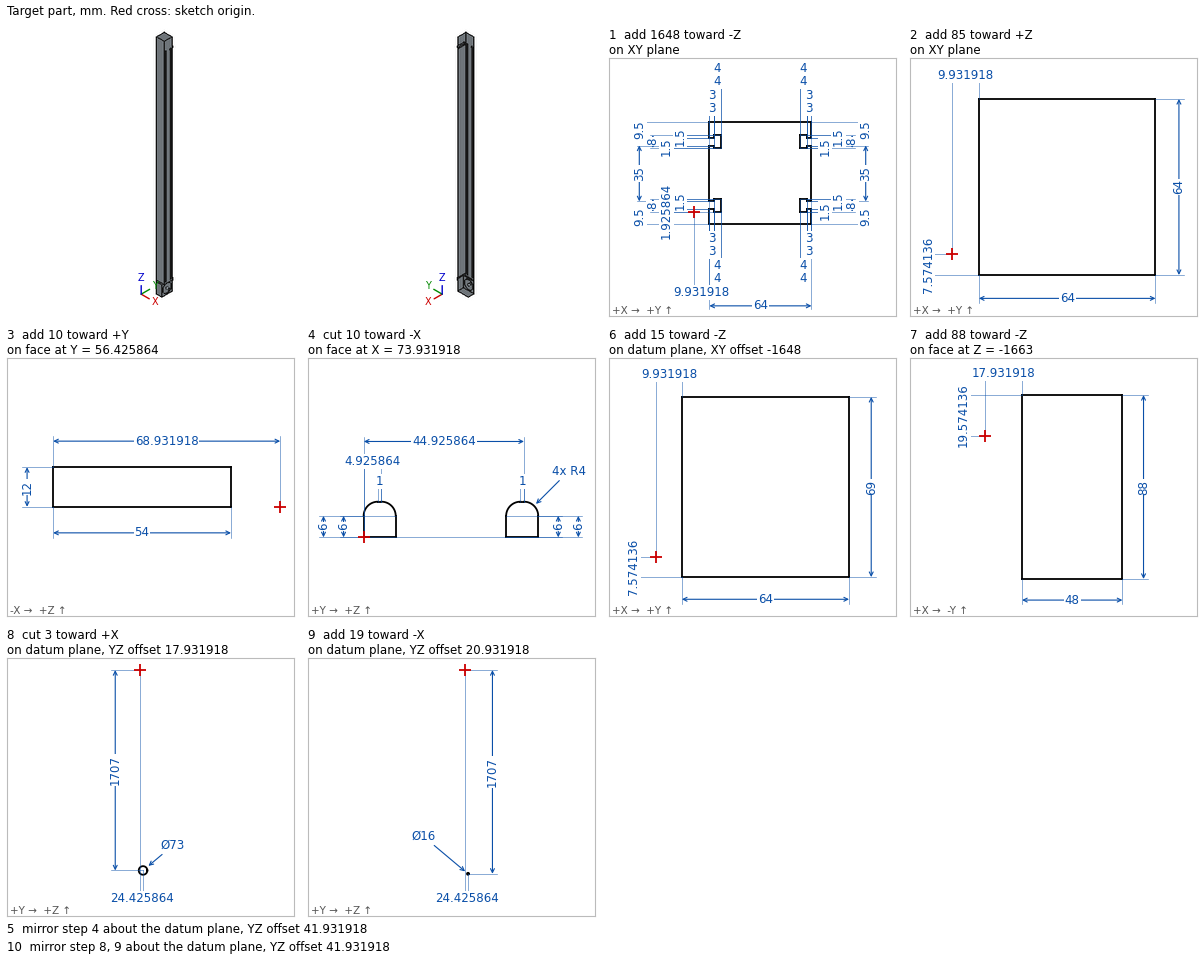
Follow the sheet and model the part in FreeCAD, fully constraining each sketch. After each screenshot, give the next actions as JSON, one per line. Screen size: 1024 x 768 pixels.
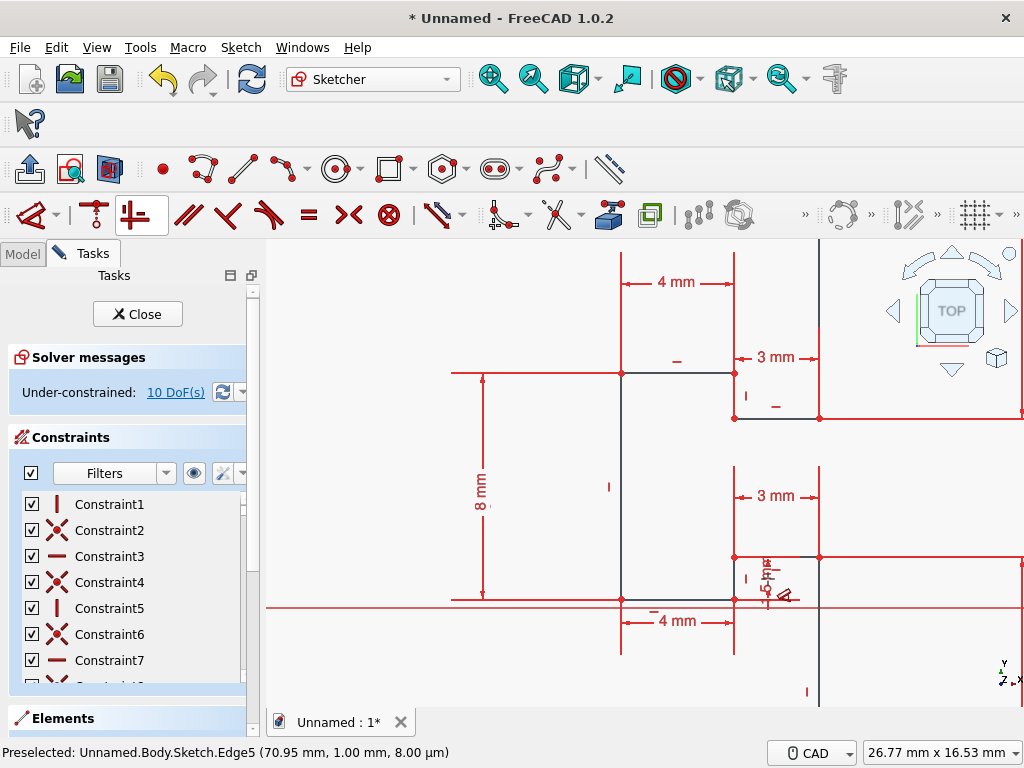
{"action": "left_click", "coordinate": [734, 387]}
{"action": "left_click", "coordinate": [768, 396]}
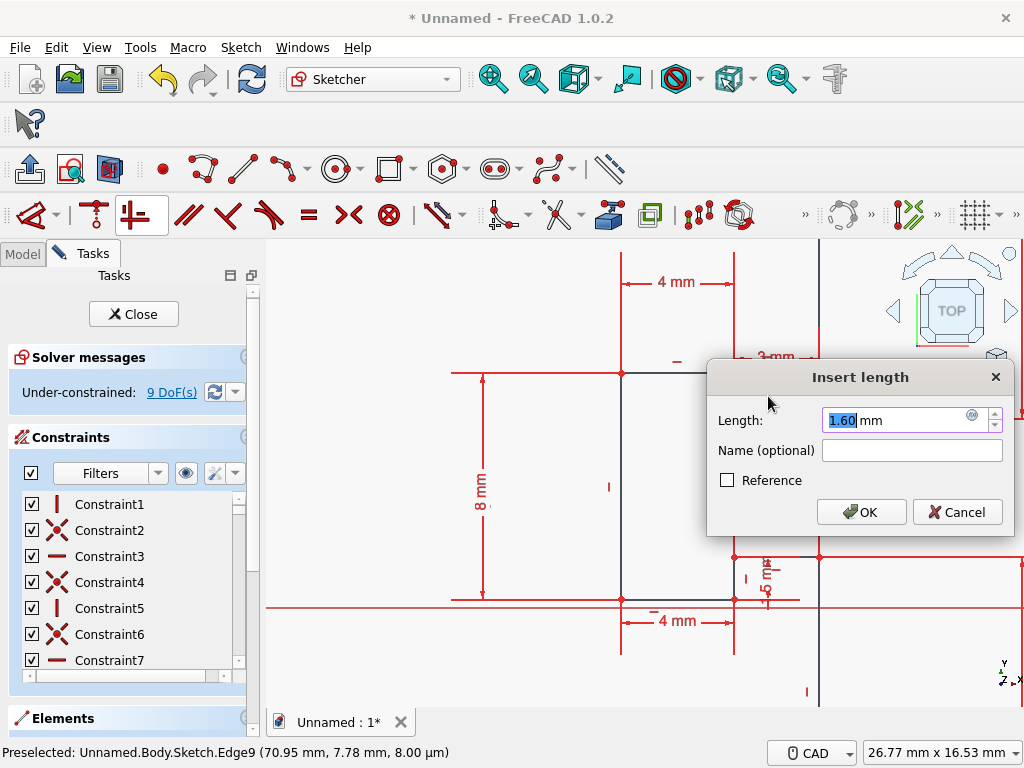
{"action": "type", "text": "1.5"}
{"action": "key", "text": "Return"}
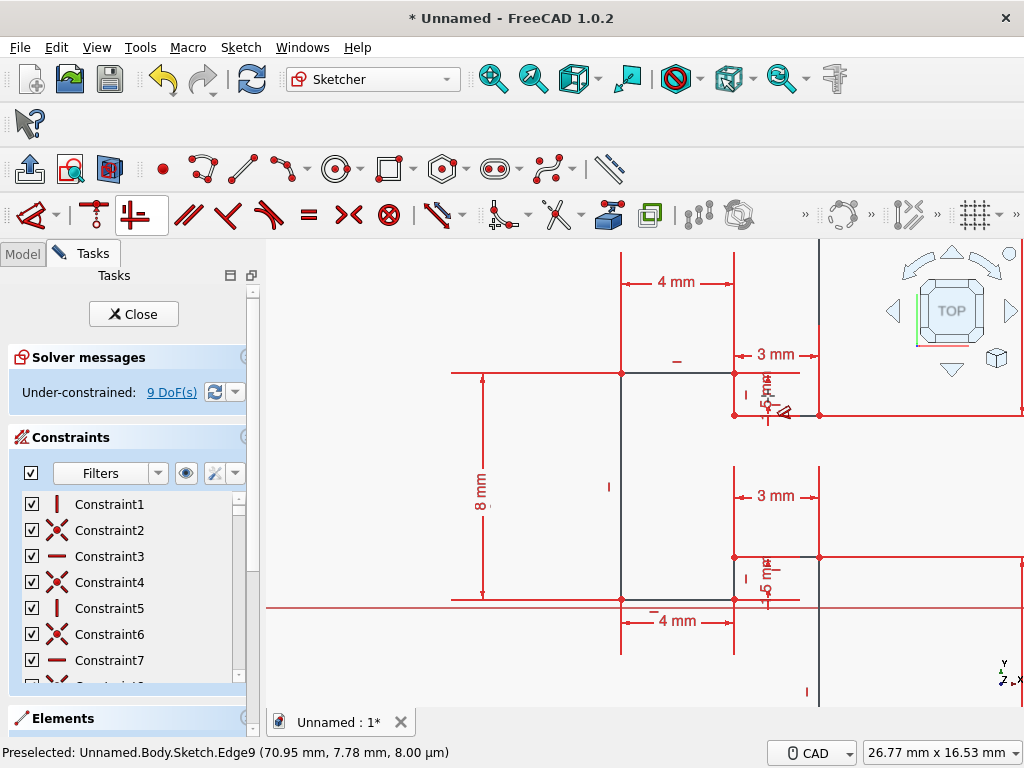
{"action": "scroll", "coordinate": [736, 583], "scroll_direction": "down", "scroll_amount": 9}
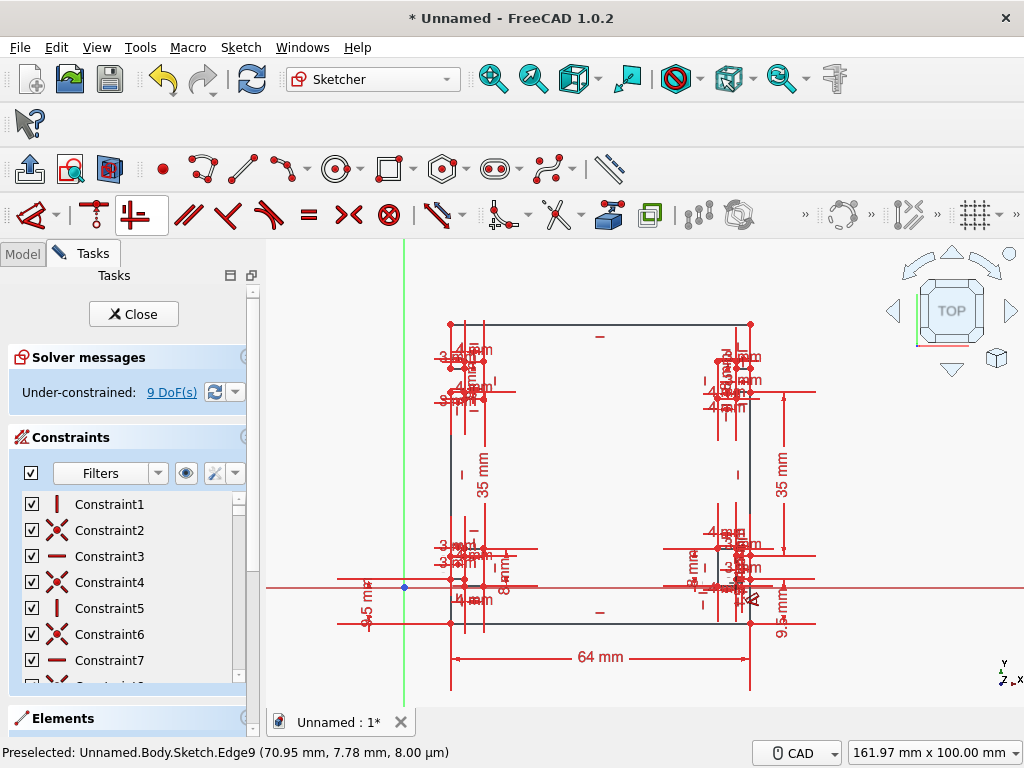
{"action": "scroll", "coordinate": [736, 394], "scroll_direction": "up", "scroll_amount": 10}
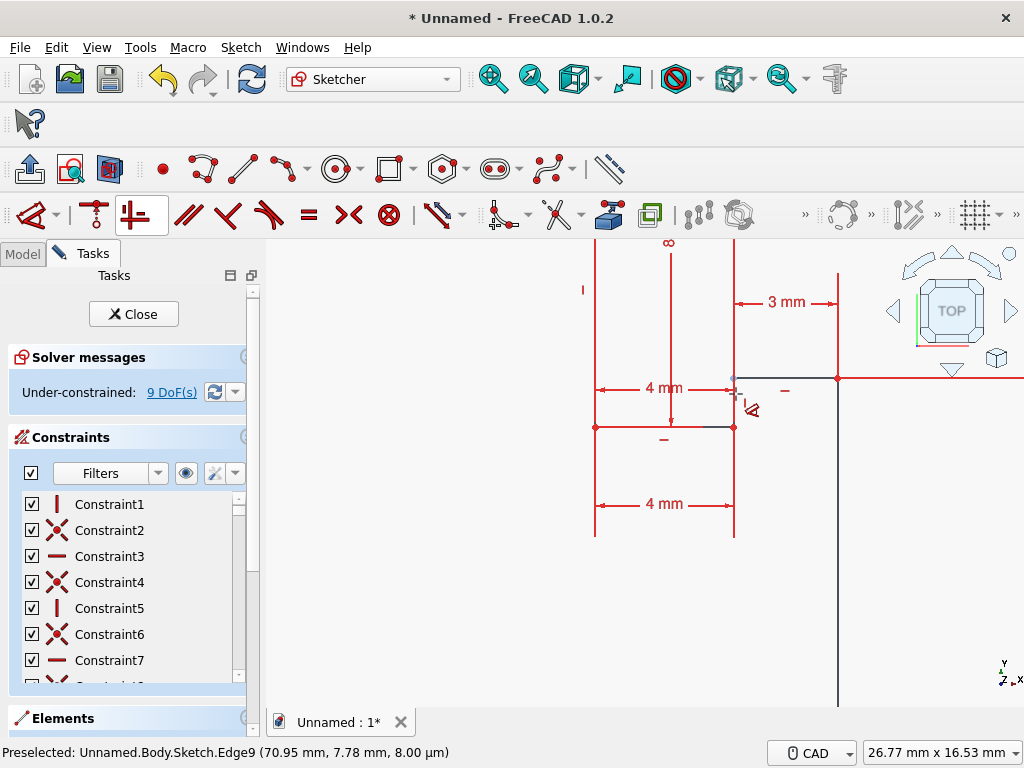
{"action": "left_click", "coordinate": [734, 393]}
{"action": "left_click", "coordinate": [768, 403]}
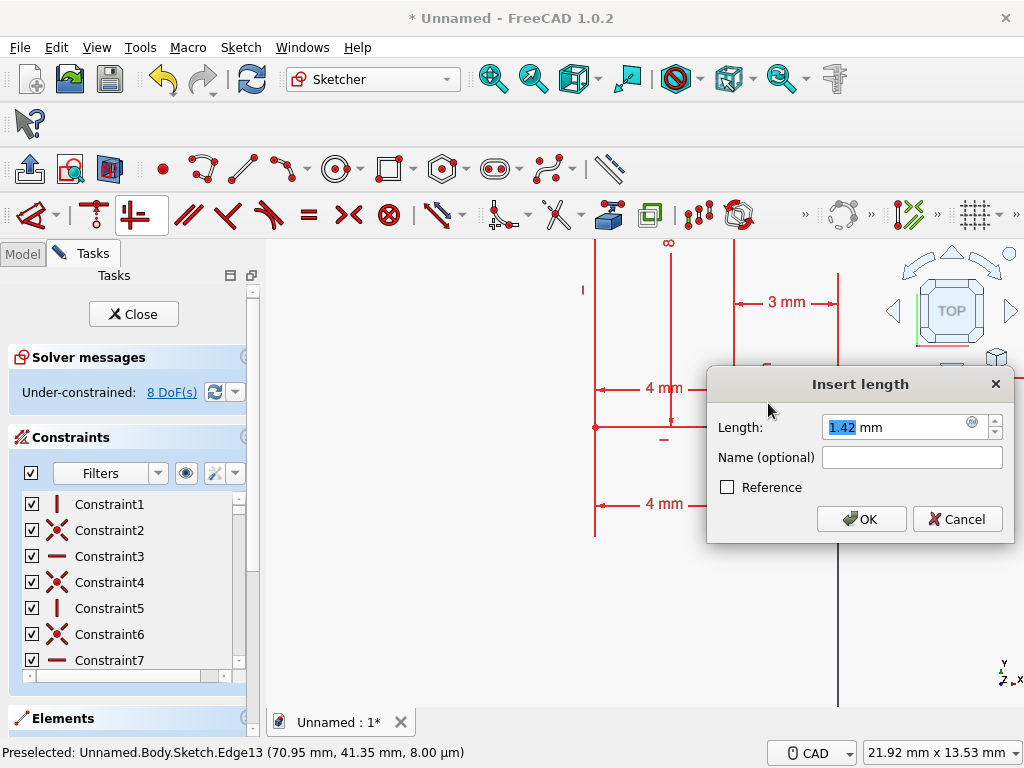
{"action": "type", "text": "1.5"}
{"action": "key", "text": "Return"}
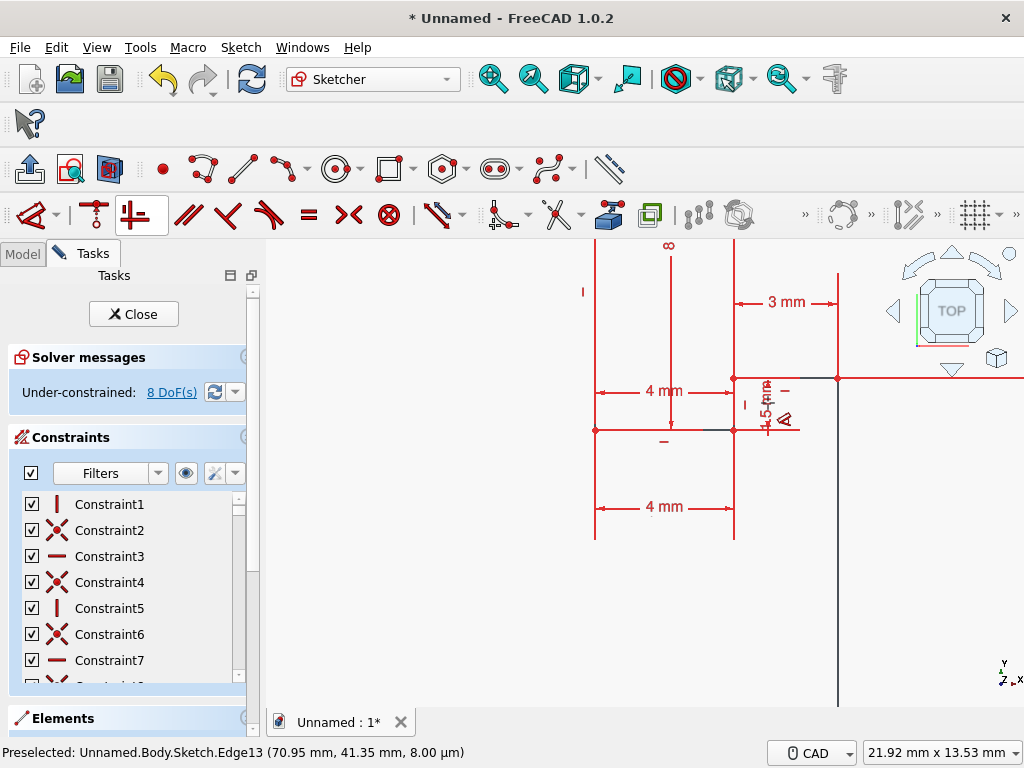
{"action": "scroll", "coordinate": [736, 394], "scroll_direction": "down", "scroll_amount": 10}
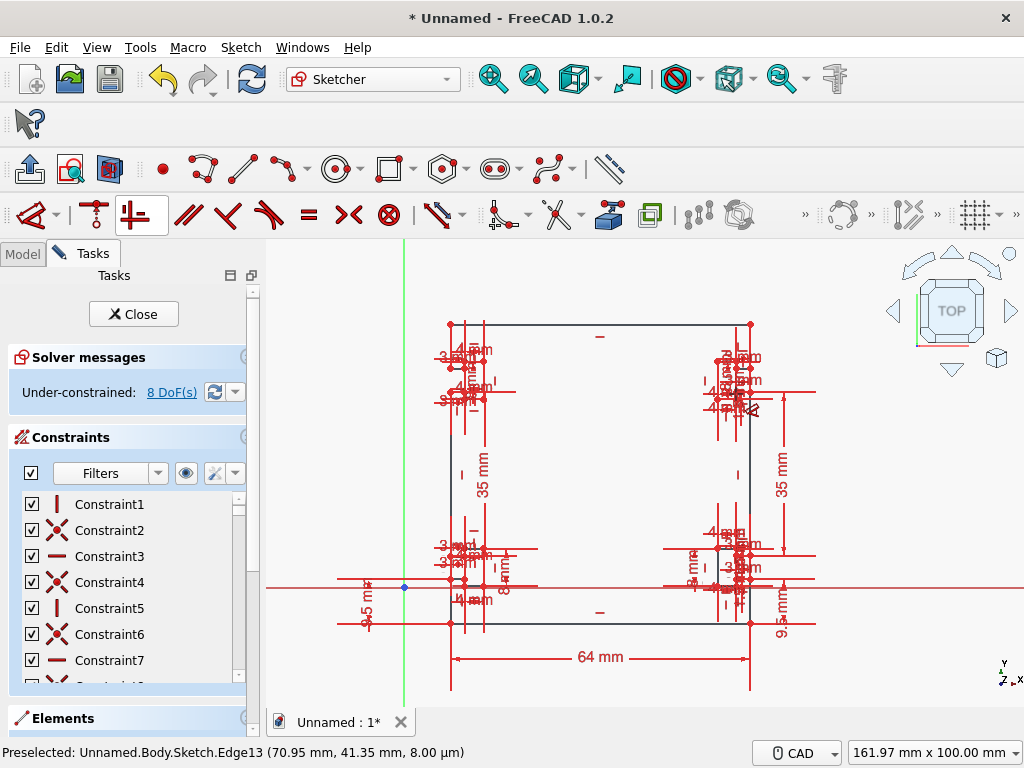
{"action": "scroll", "coordinate": [736, 364], "scroll_direction": "up", "scroll_amount": 10}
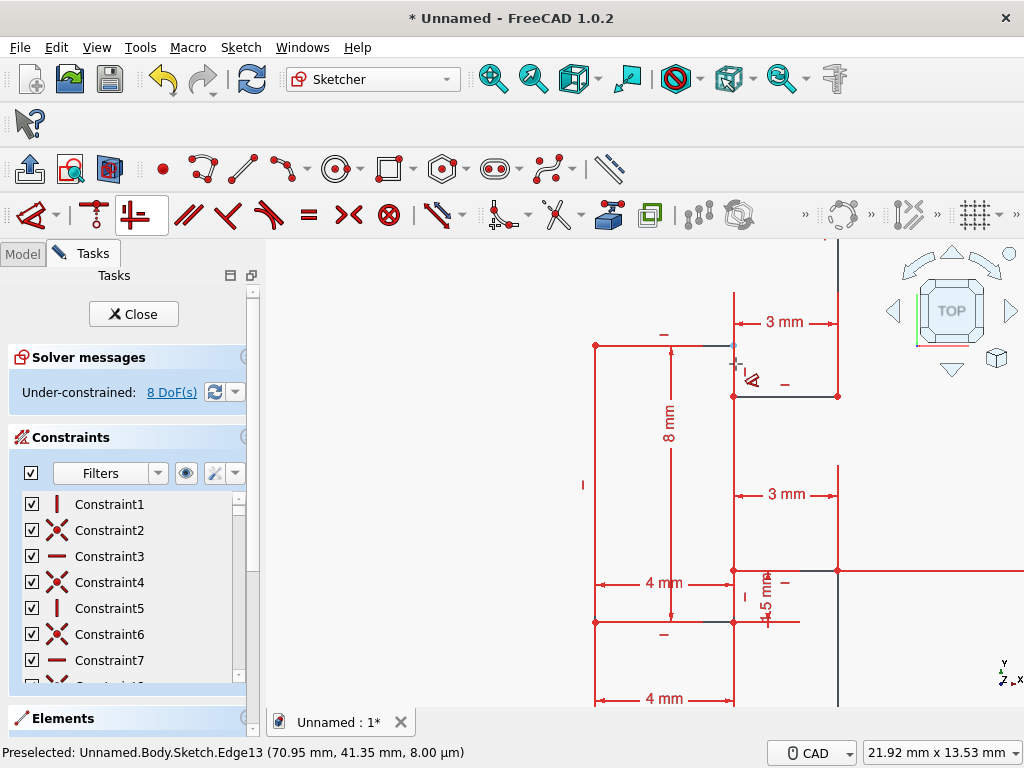
{"action": "left_click", "coordinate": [734, 361]}
{"action": "left_click", "coordinate": [768, 371]}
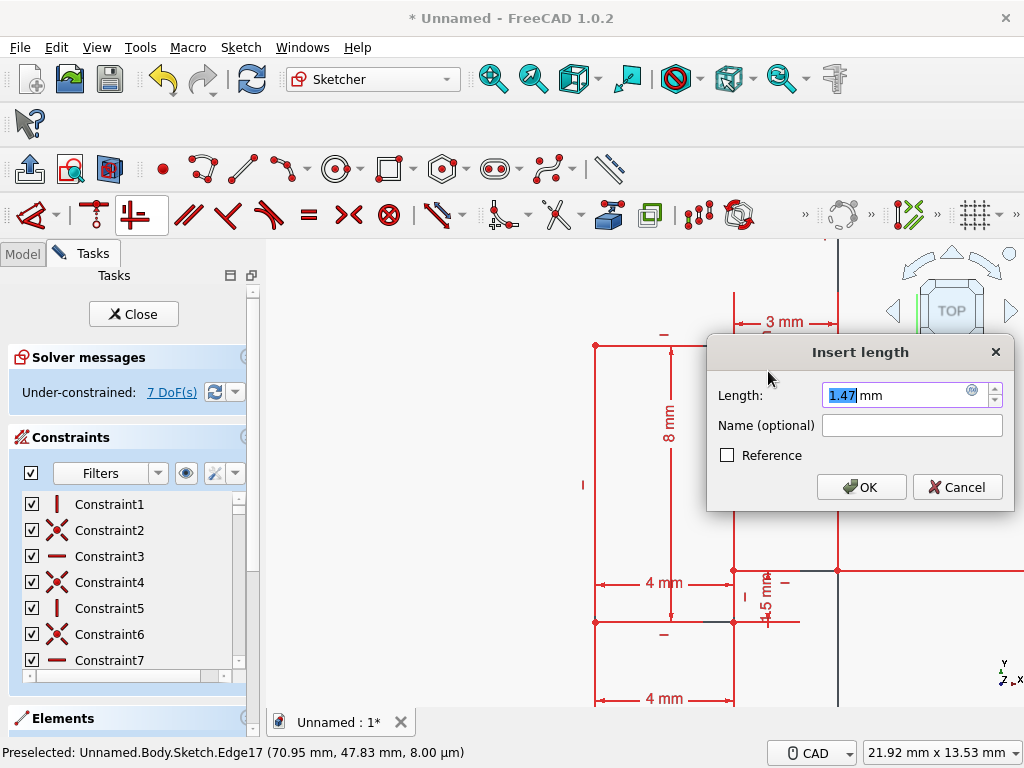
{"action": "type", "text": "1.5"}
{"action": "key", "text": "Return"}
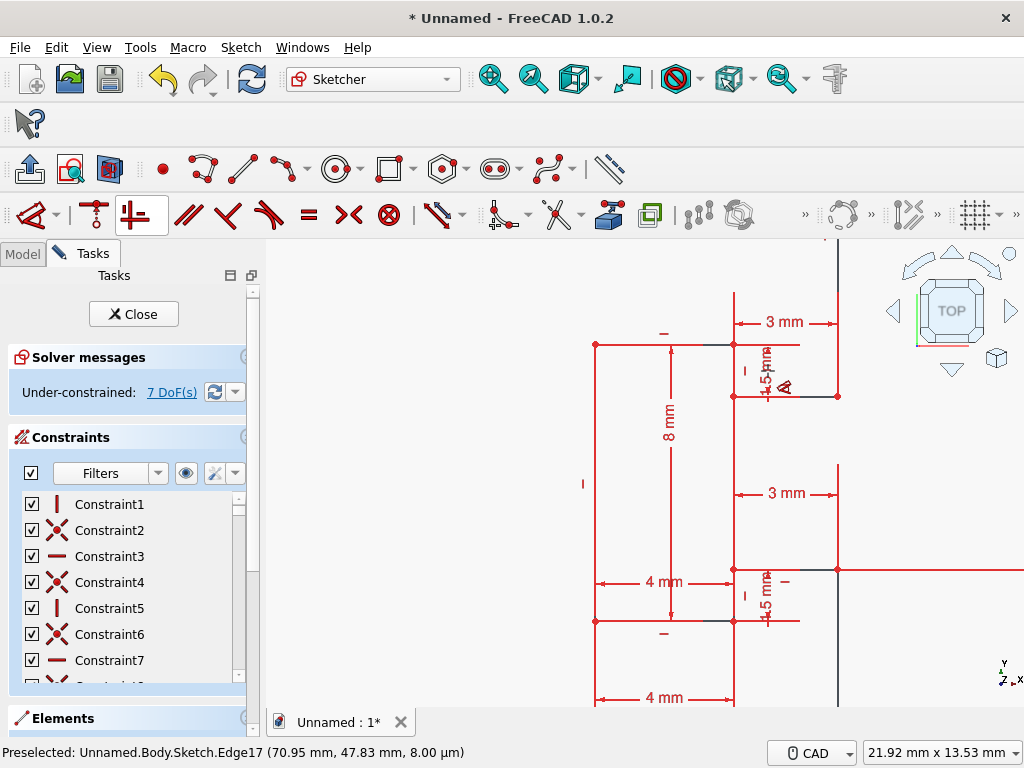
{"action": "scroll", "coordinate": [736, 364], "scroll_direction": "down", "scroll_amount": 10}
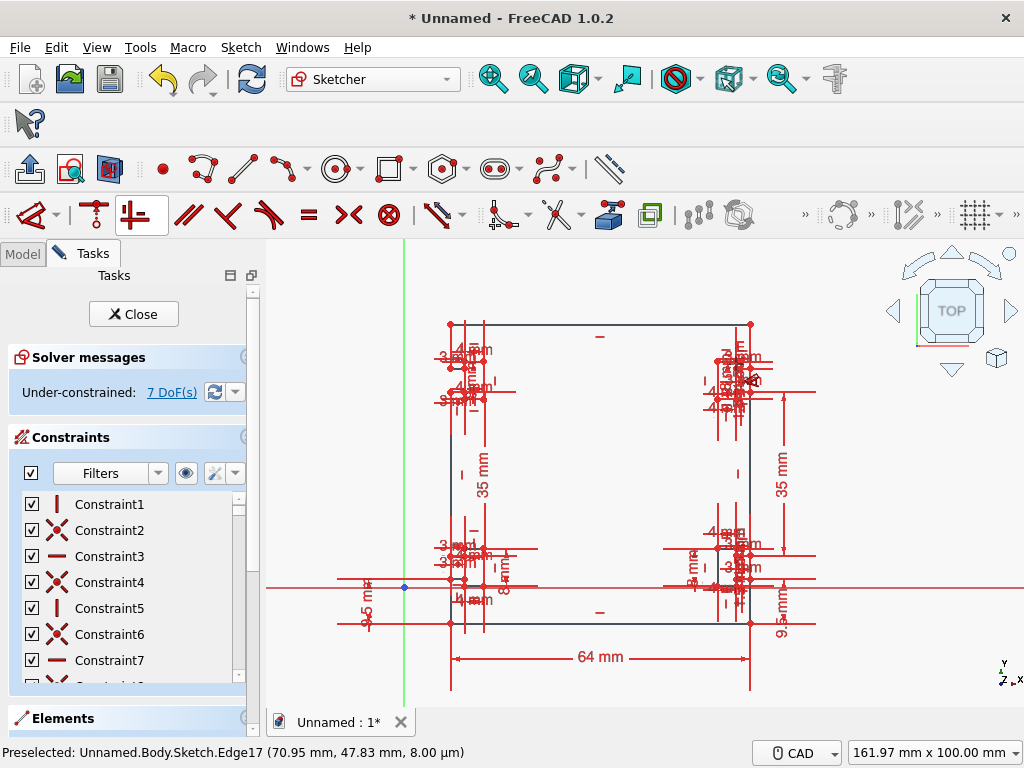
{"action": "left_click", "coordinate": [750, 356]}
{"action": "left_click", "coordinate": [784, 337]}